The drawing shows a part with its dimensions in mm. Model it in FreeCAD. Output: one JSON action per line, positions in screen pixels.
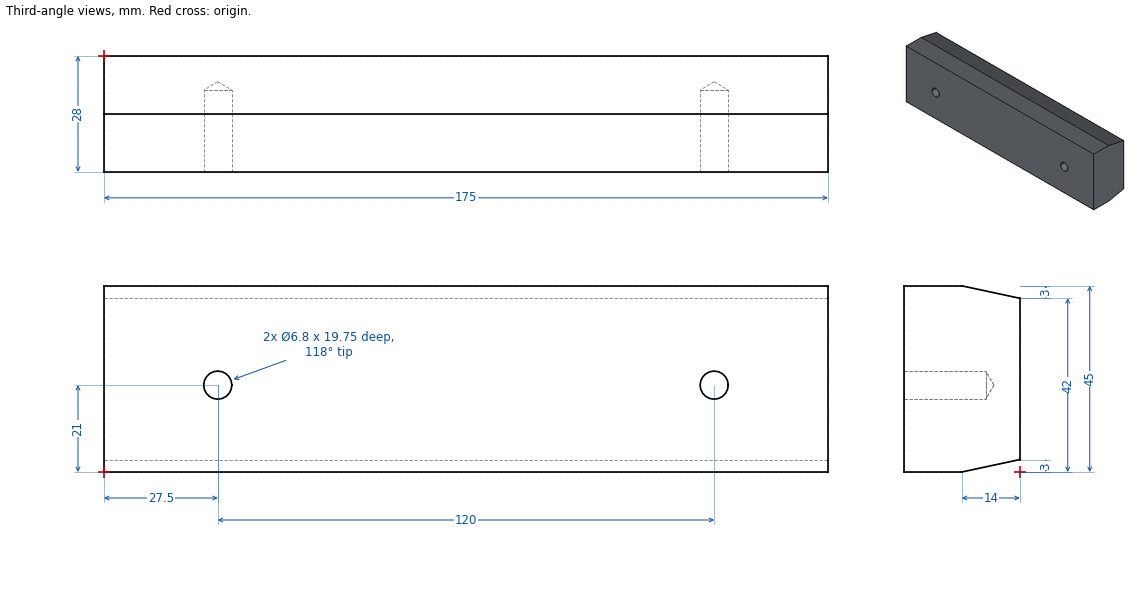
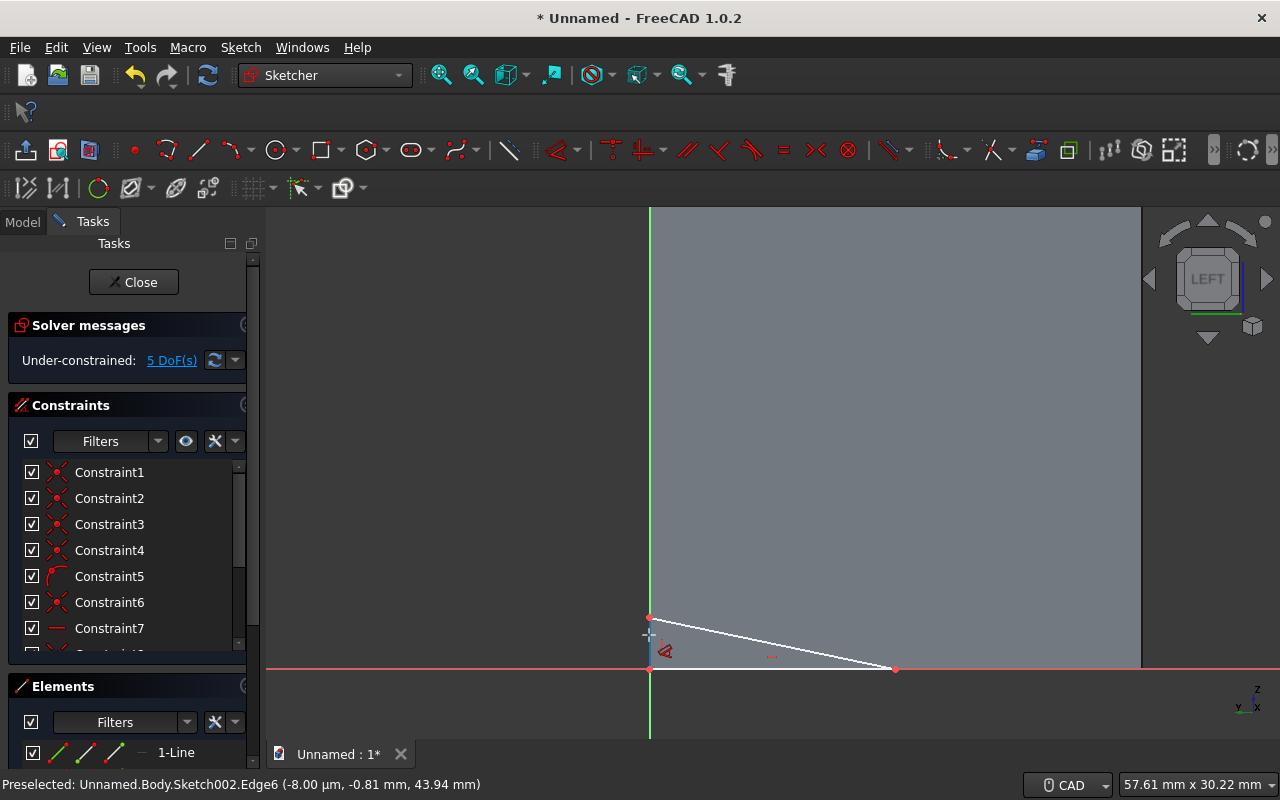
{"action": "left_click", "coordinate": [650, 633]}
{"action": "left_click", "coordinate": [616, 644]}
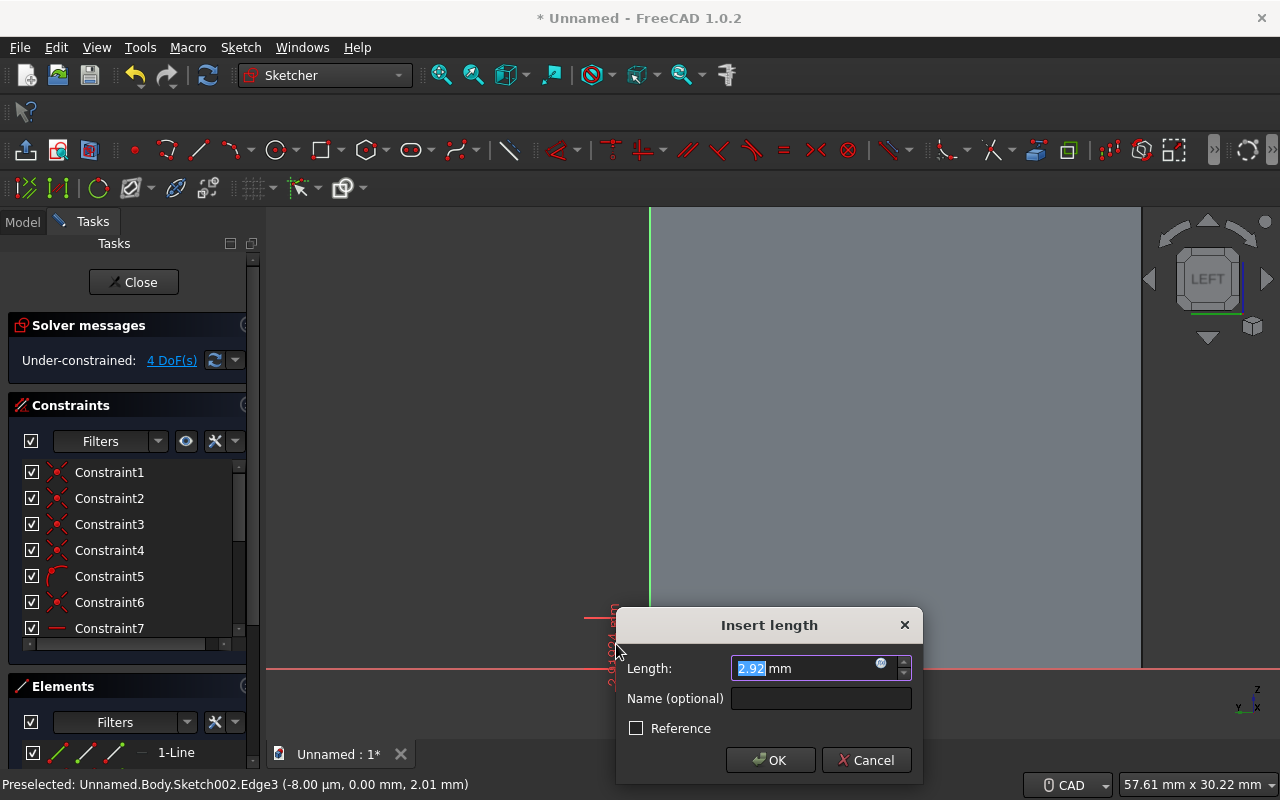
{"action": "type", "text": "3"}
{"action": "key", "text": "Return"}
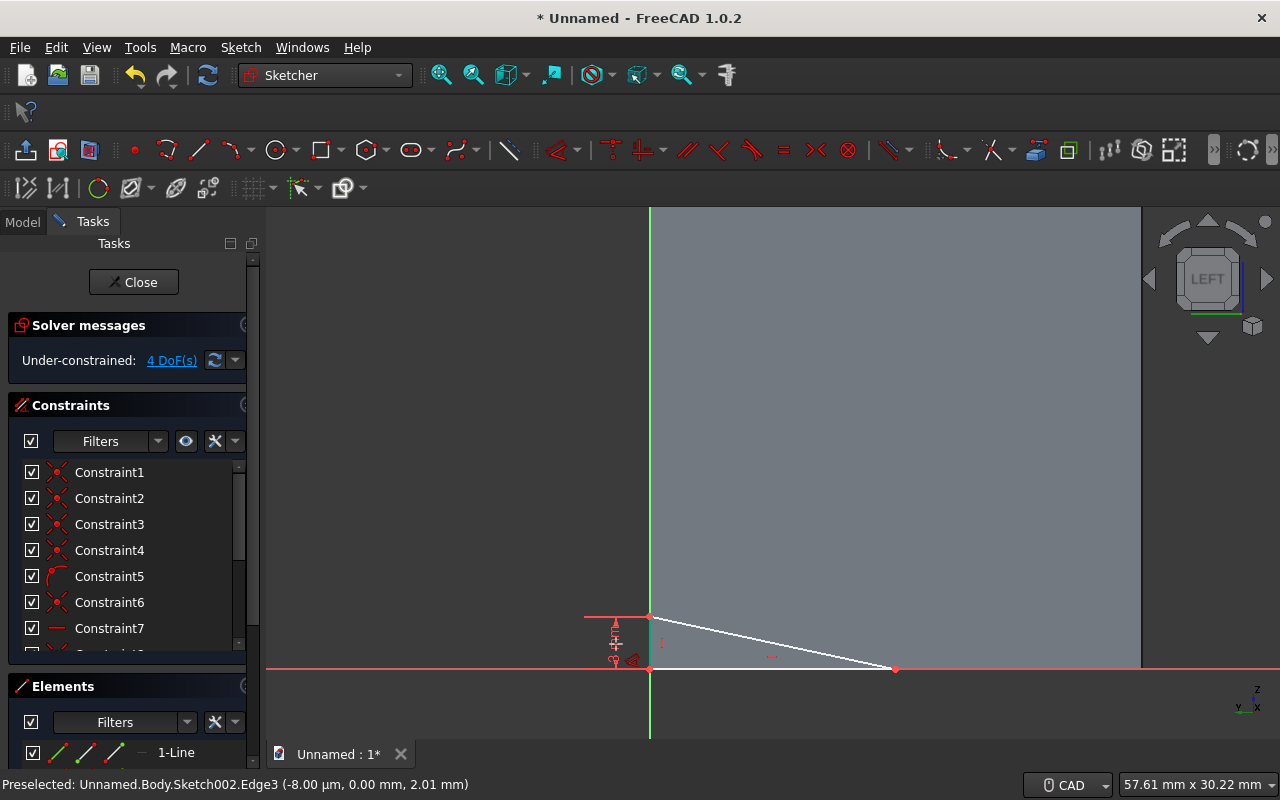
{"action": "scroll", "coordinate": [649, 636], "scroll_direction": "down", "scroll_amount": 4}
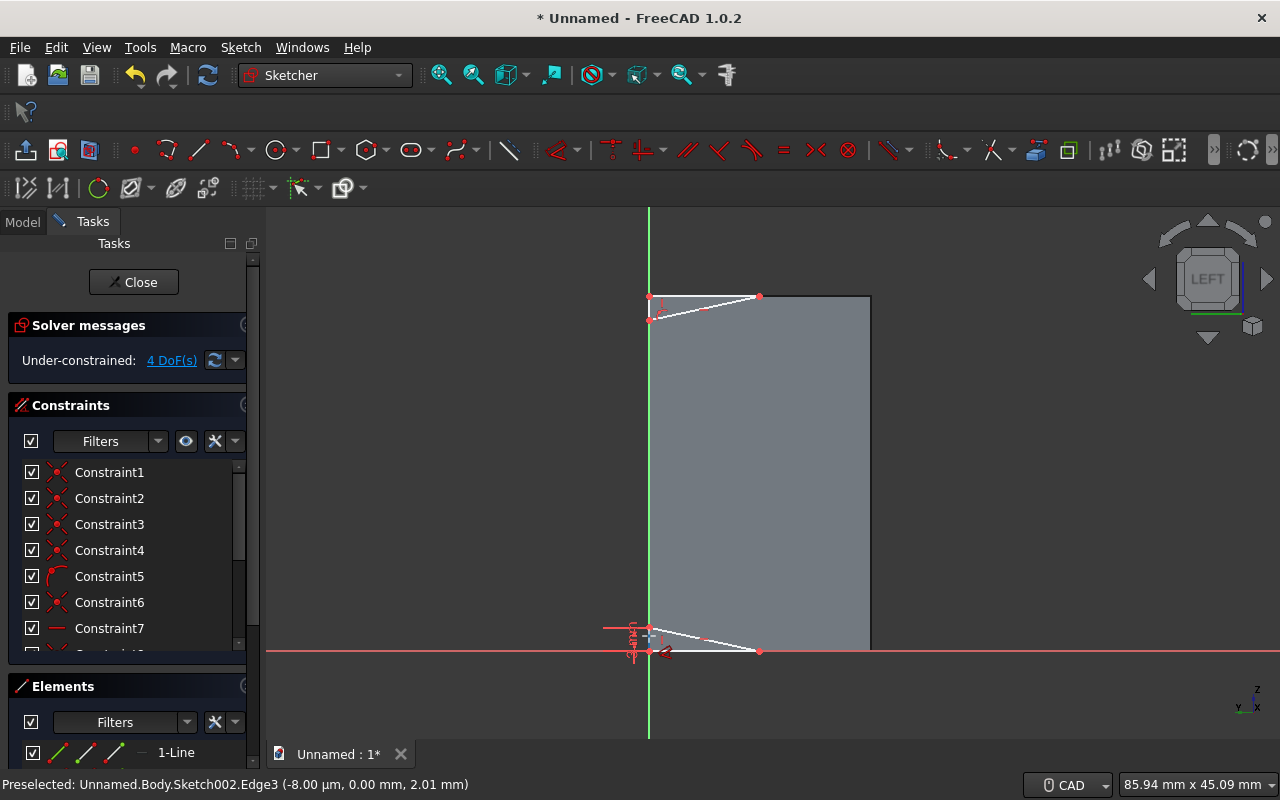
{"action": "scroll", "coordinate": [649, 304], "scroll_direction": "up", "scroll_amount": 4}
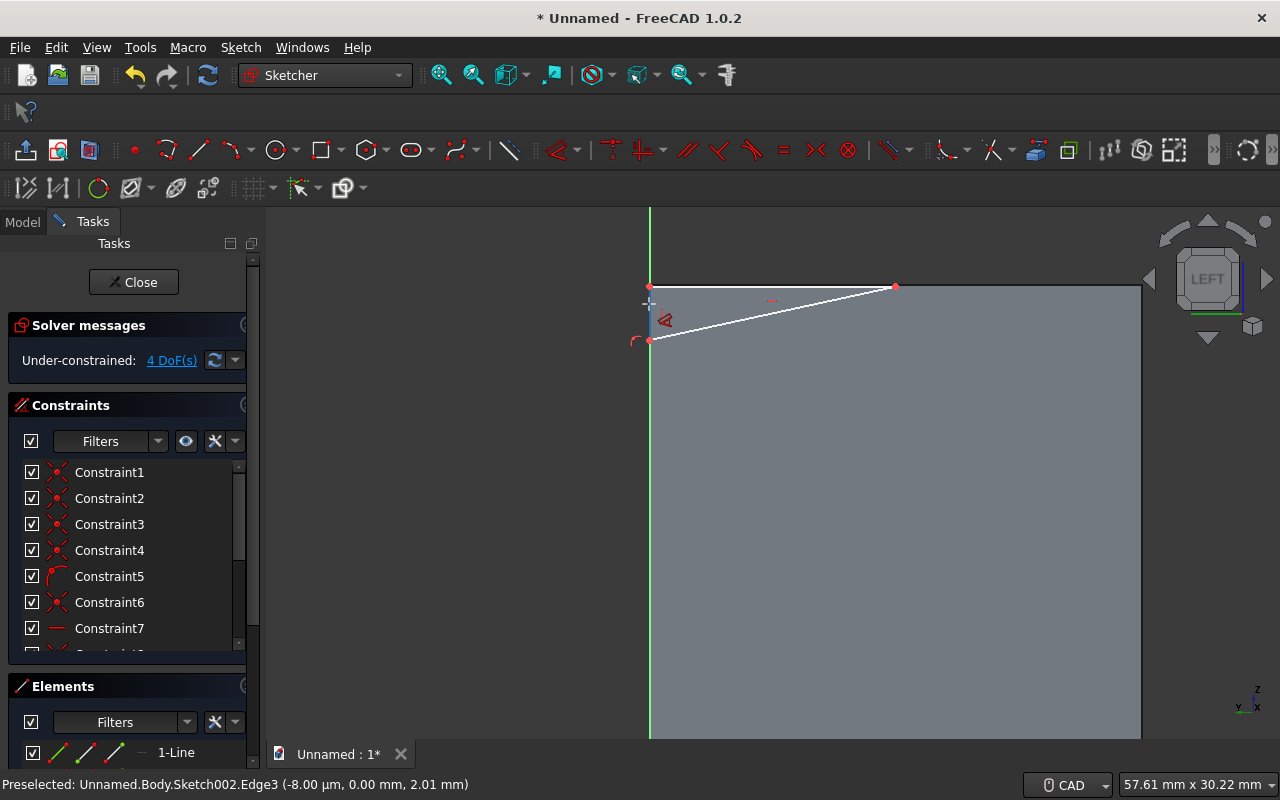
{"action": "left_click", "coordinate": [650, 303]}
{"action": "left_click", "coordinate": [616, 313]}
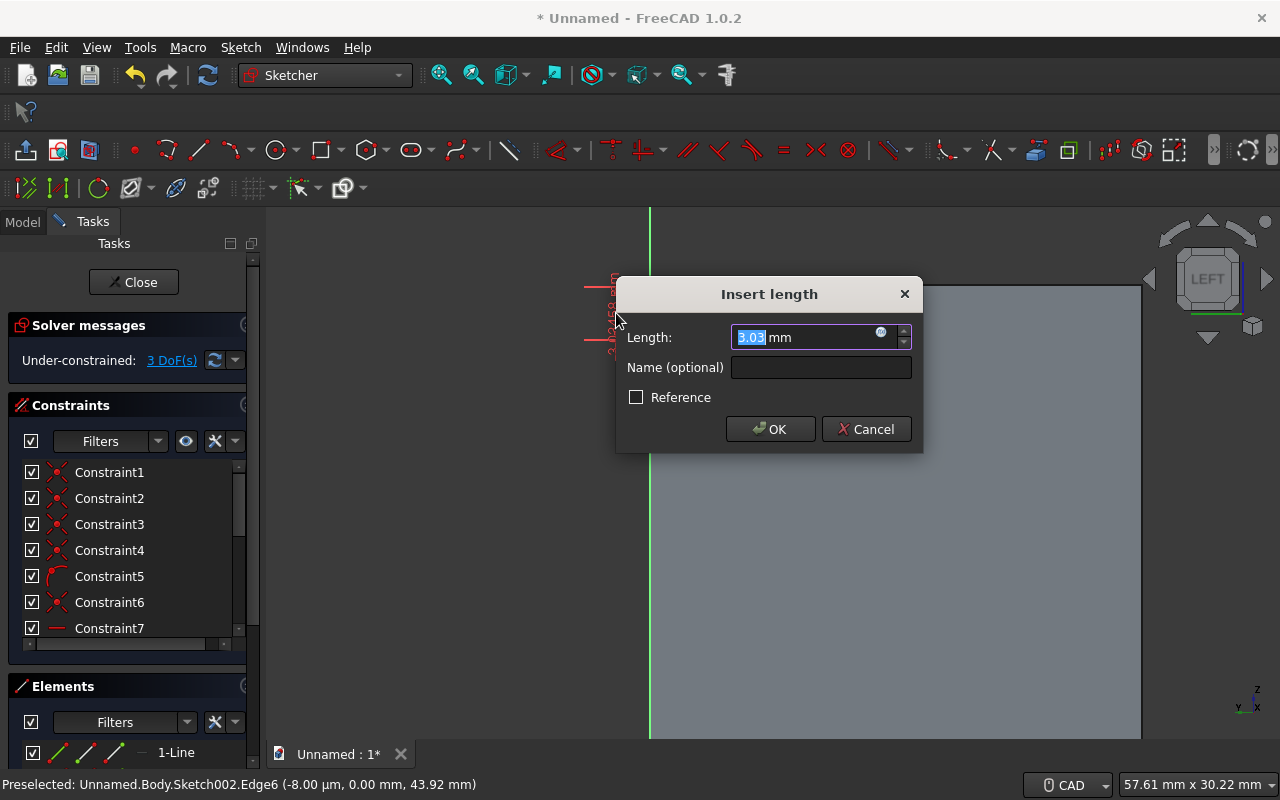
{"action": "type", "text": "3"}
{"action": "key", "text": "Return"}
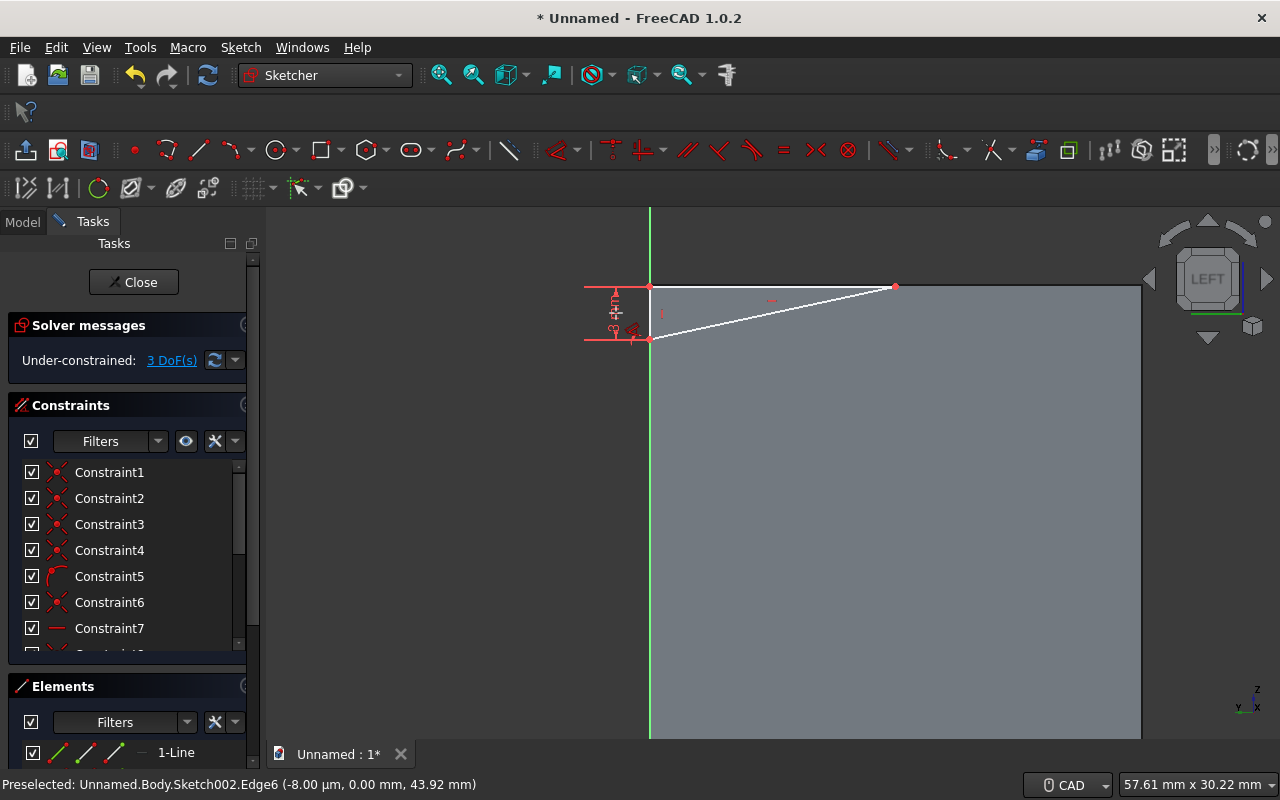
{"action": "scroll", "coordinate": [649, 303], "scroll_direction": "down", "scroll_amount": 4}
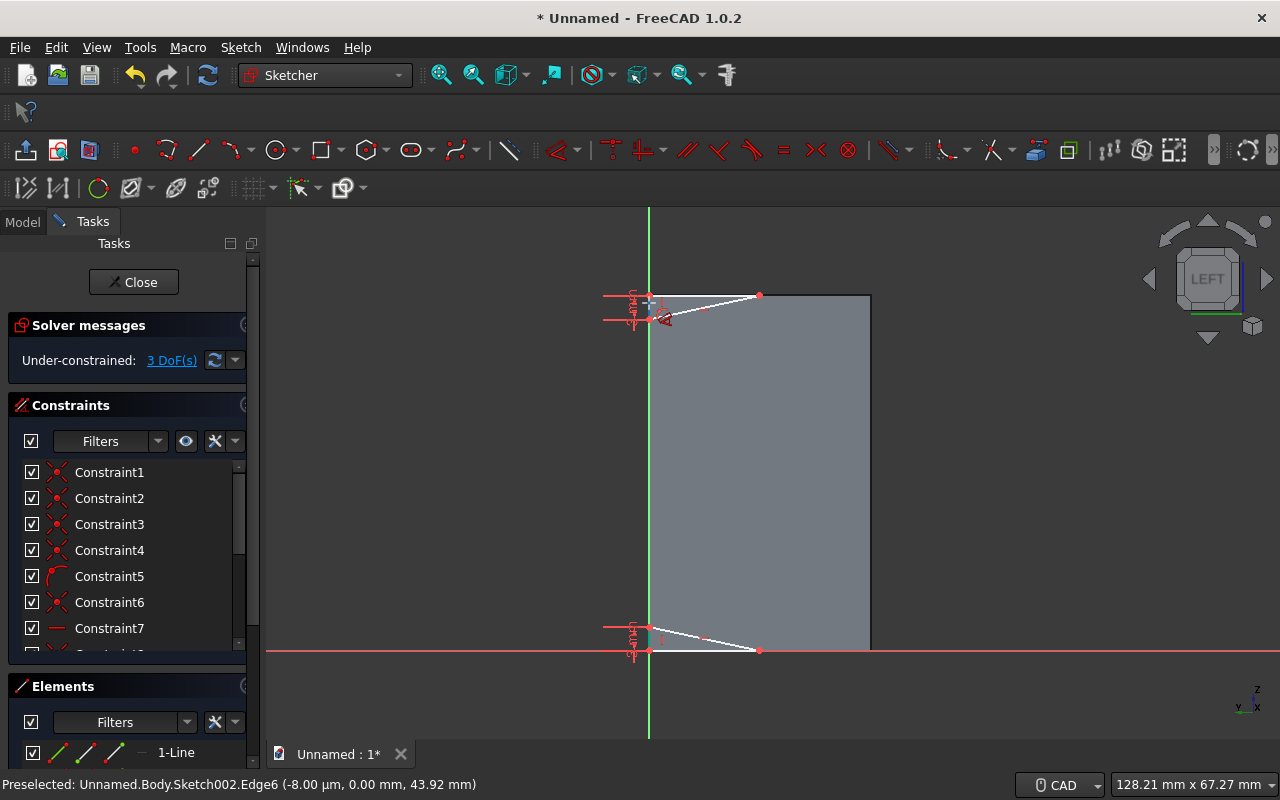
{"action": "left_click", "coordinate": [683, 651]}
{"action": "left_click", "coordinate": [705, 685]}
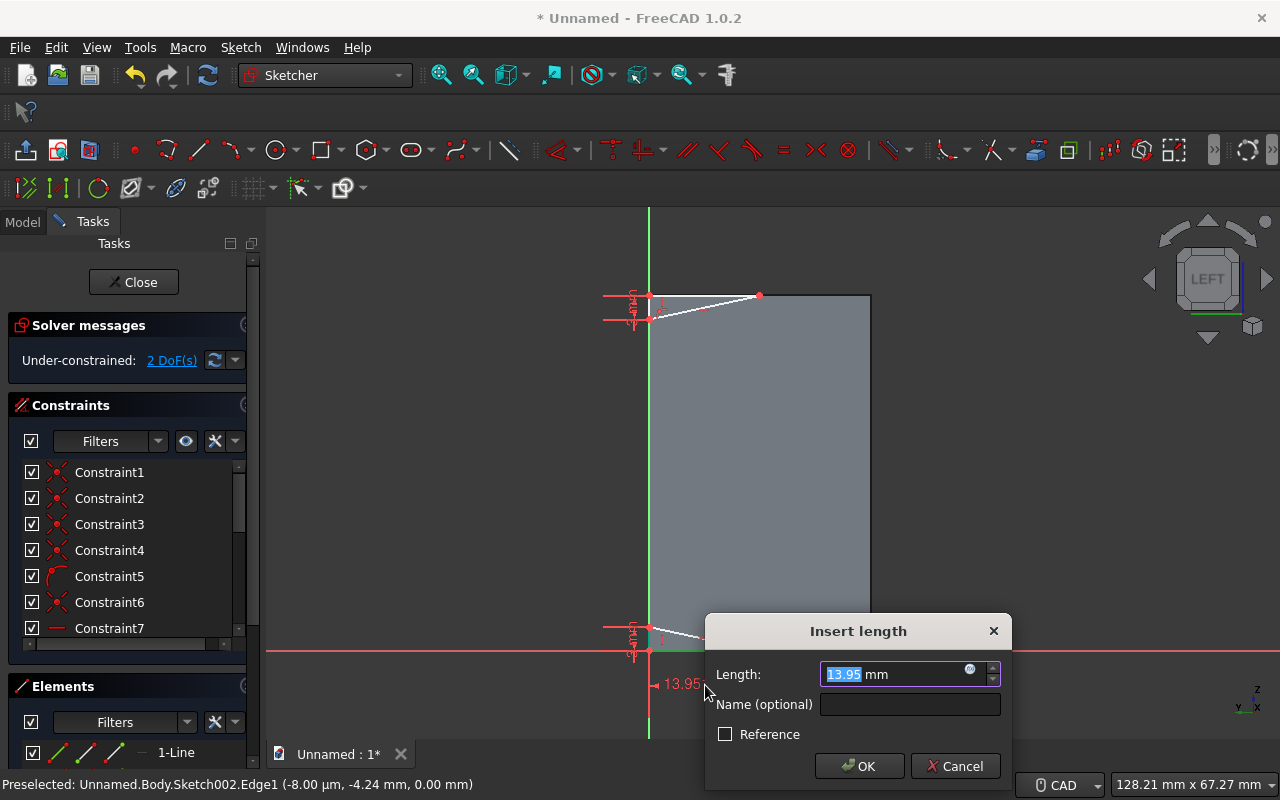
{"action": "type", "text": "14"}
{"action": "key", "text": "Return"}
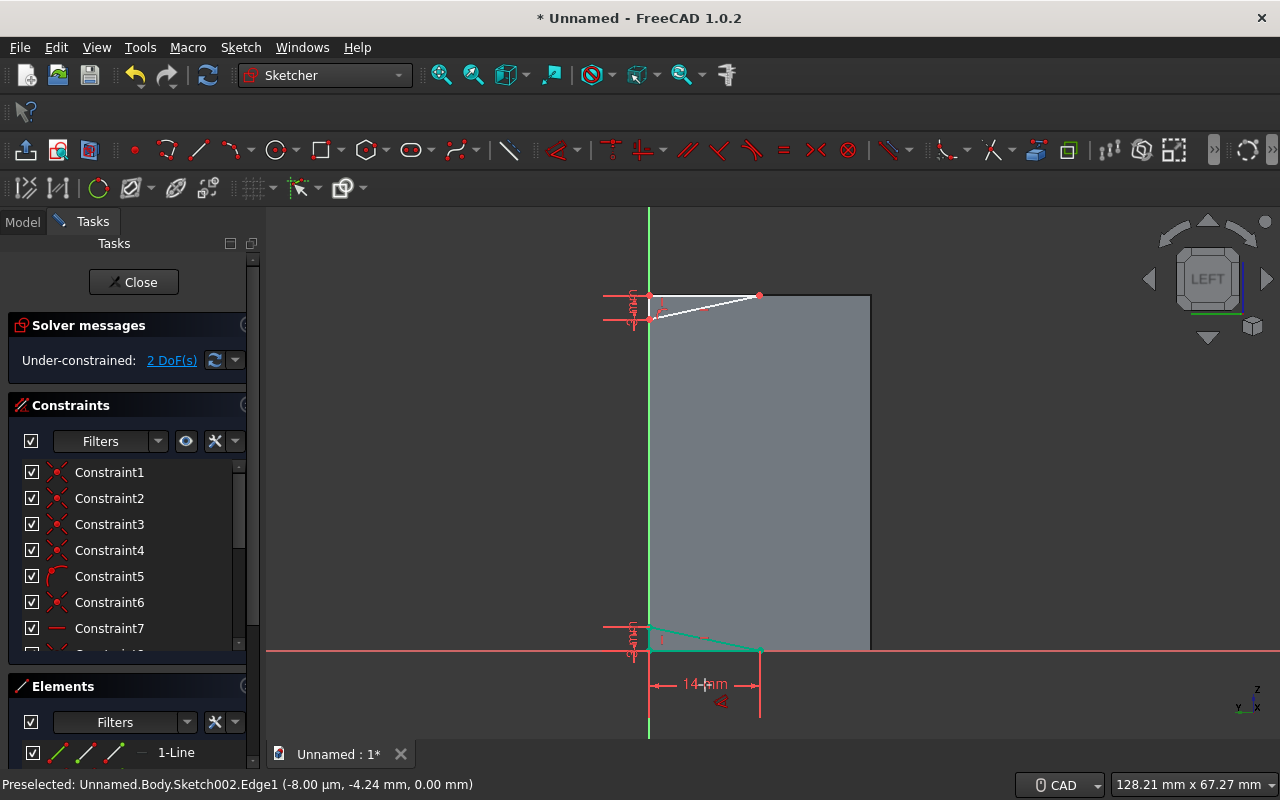
{"action": "left_click", "coordinate": [683, 296]}
{"action": "left_click", "coordinate": [705, 262]}